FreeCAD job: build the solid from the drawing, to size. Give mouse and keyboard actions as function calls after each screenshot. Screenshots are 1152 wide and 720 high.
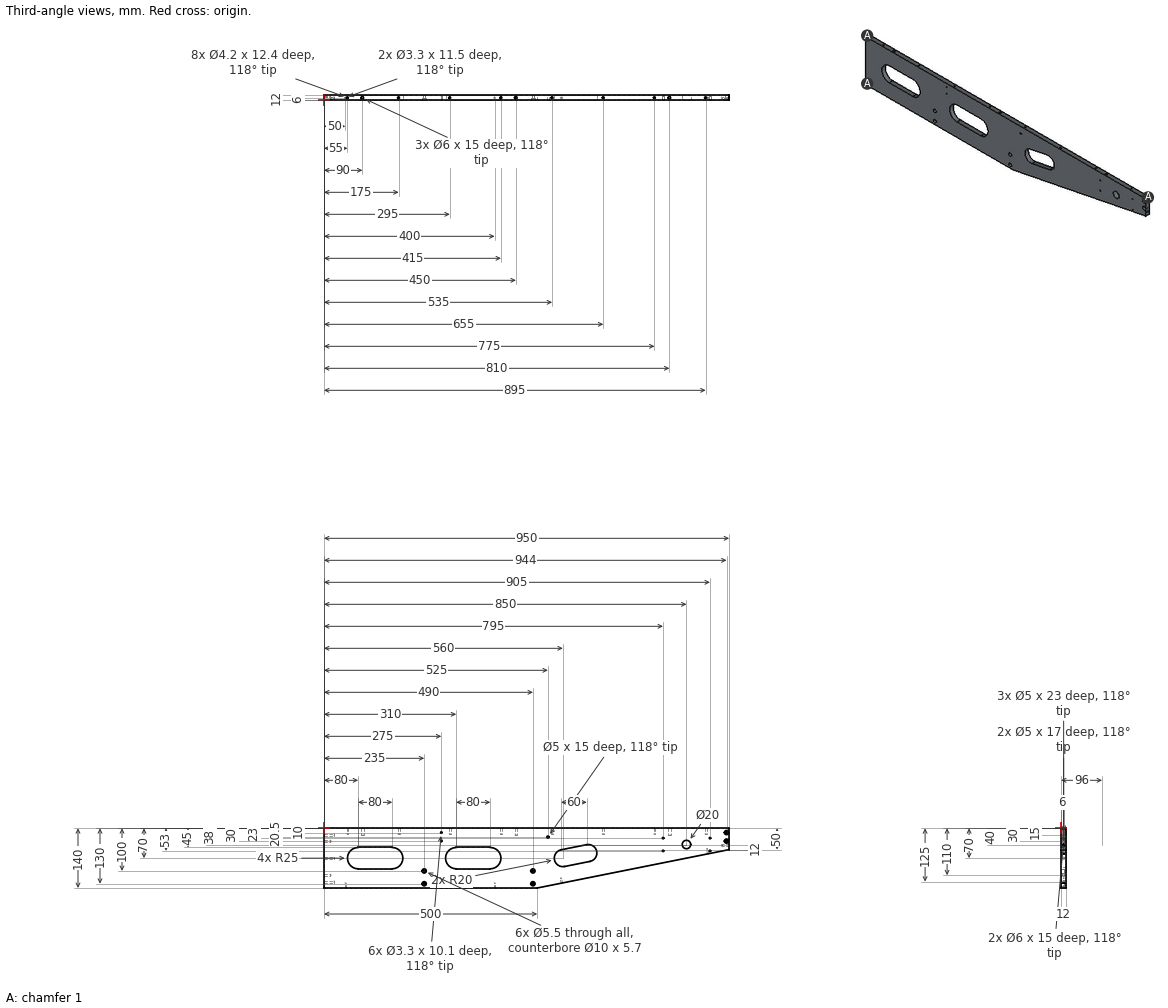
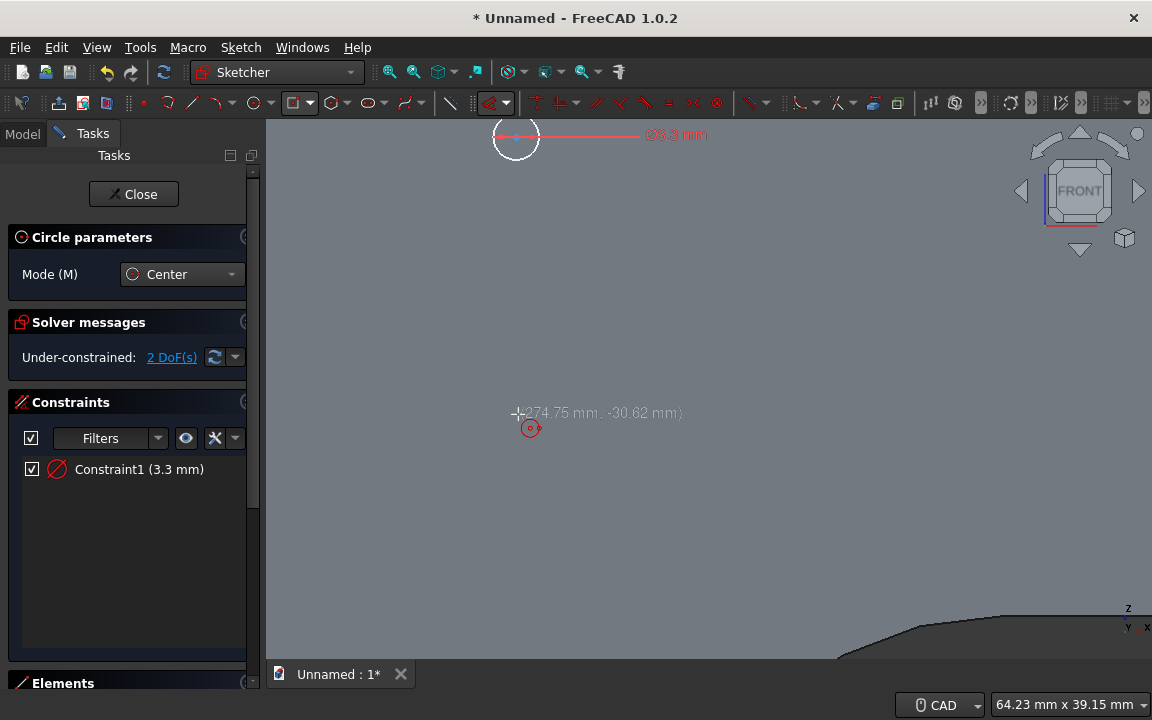
scroll(518, 390, down, 15)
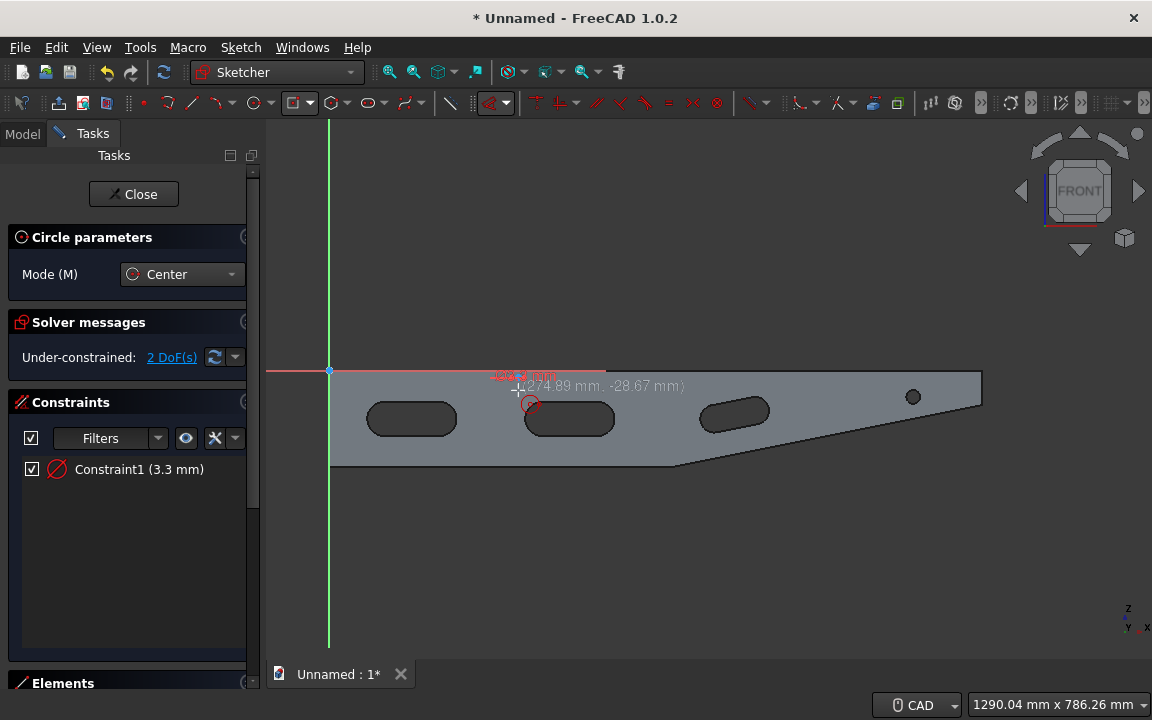
scroll(518, 391, up, 2)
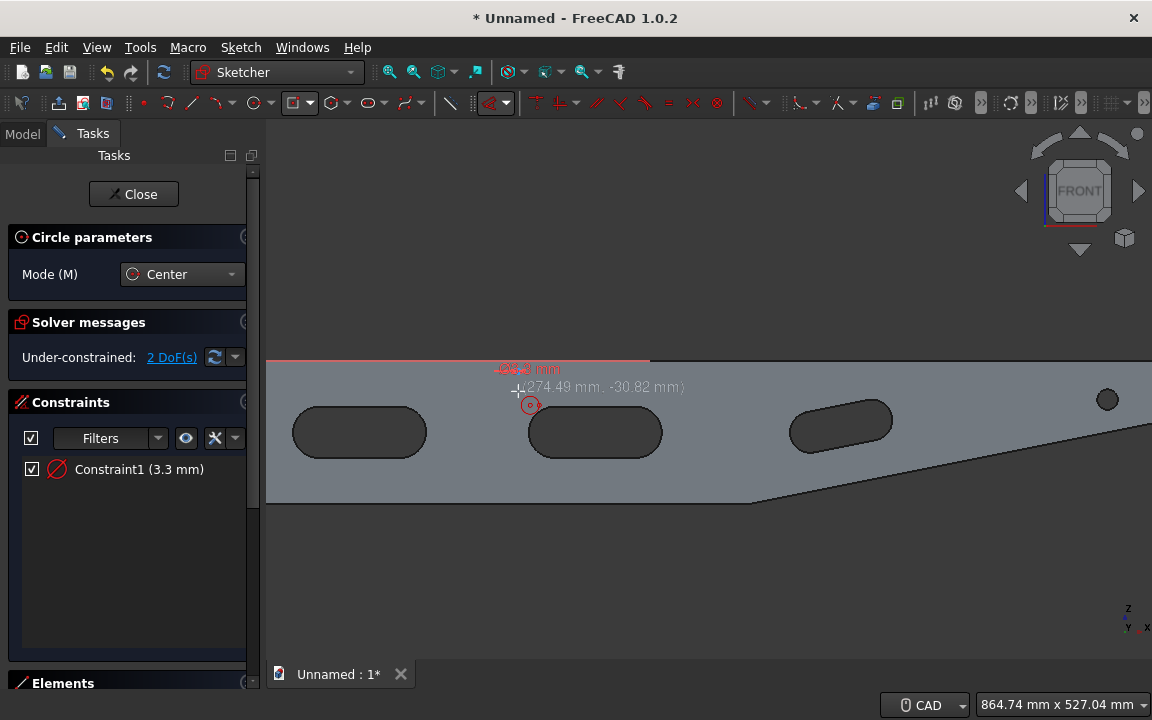
click(518, 391)
move(520, 390)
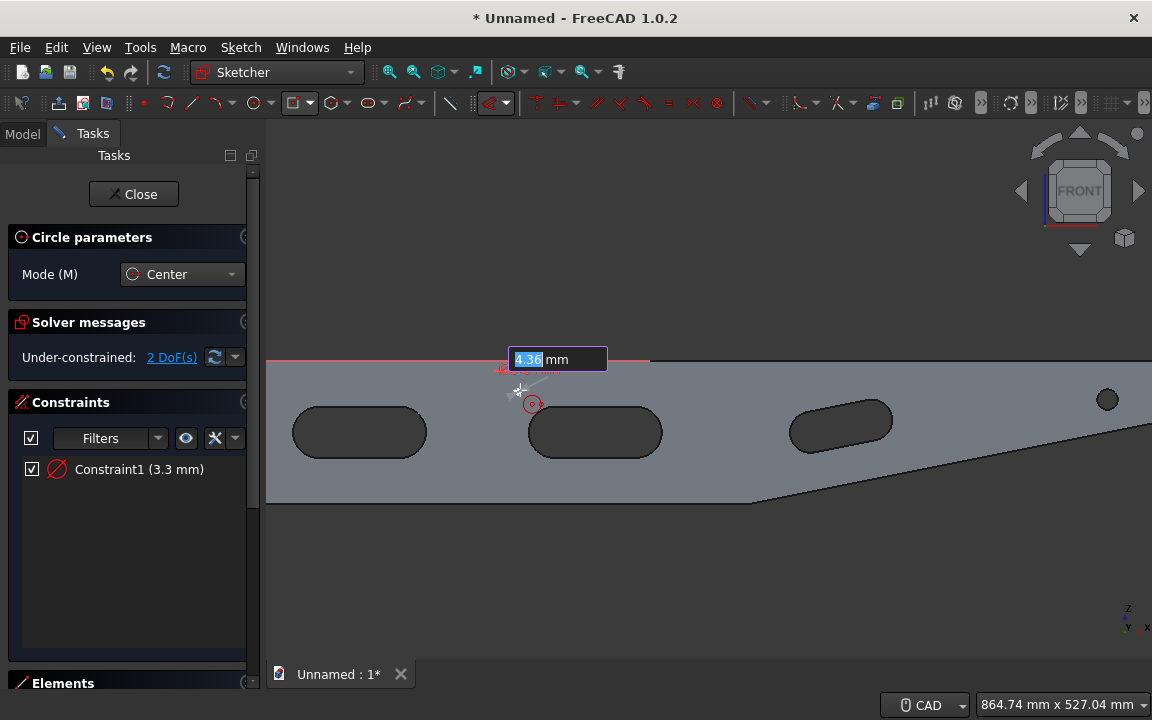
text(3.3)
key(Return)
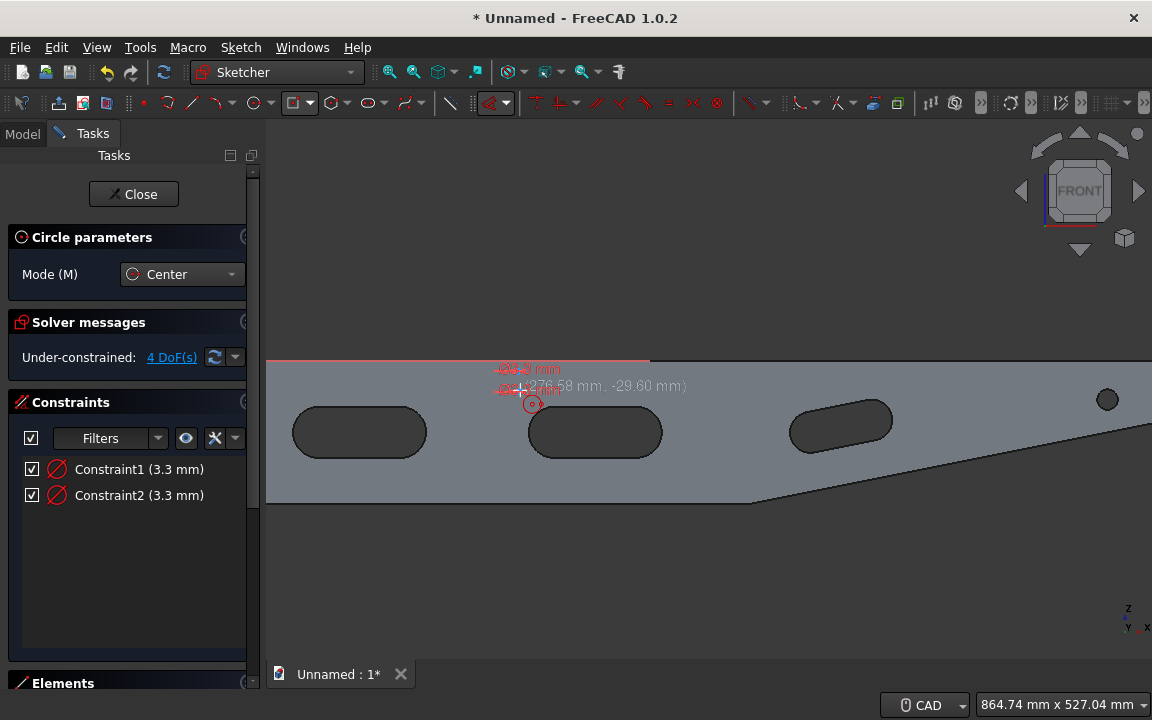
scroll(567, 389, down, 3)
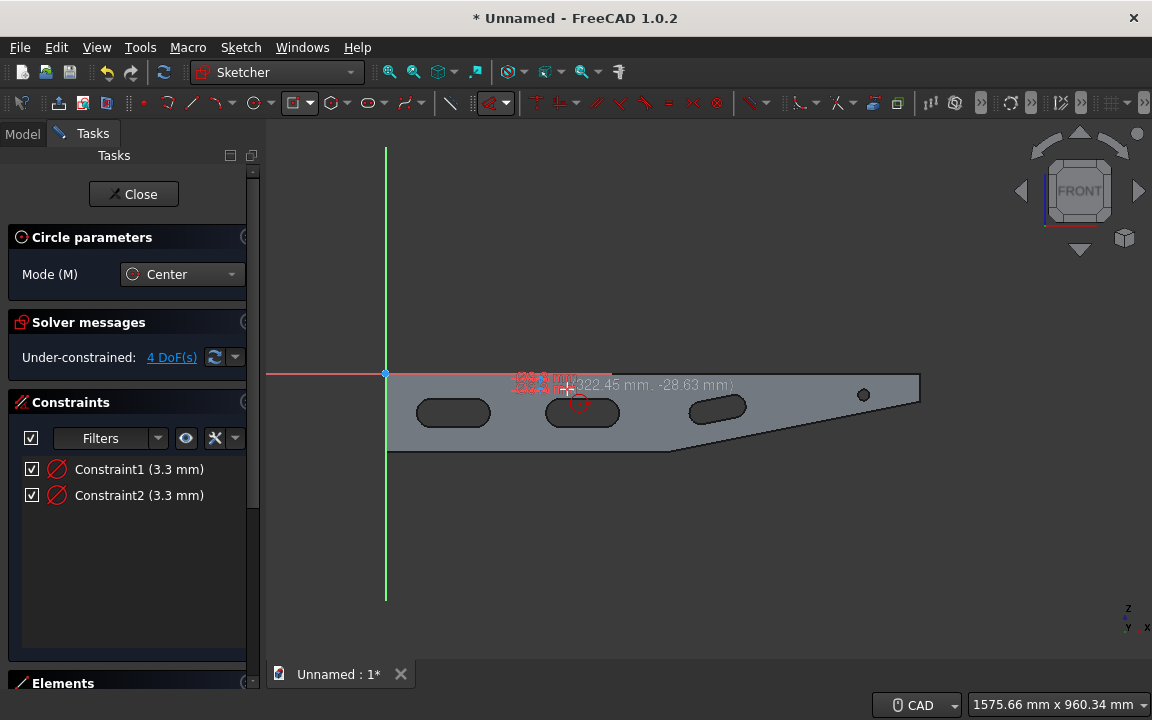
scroll(833, 387, up, 16)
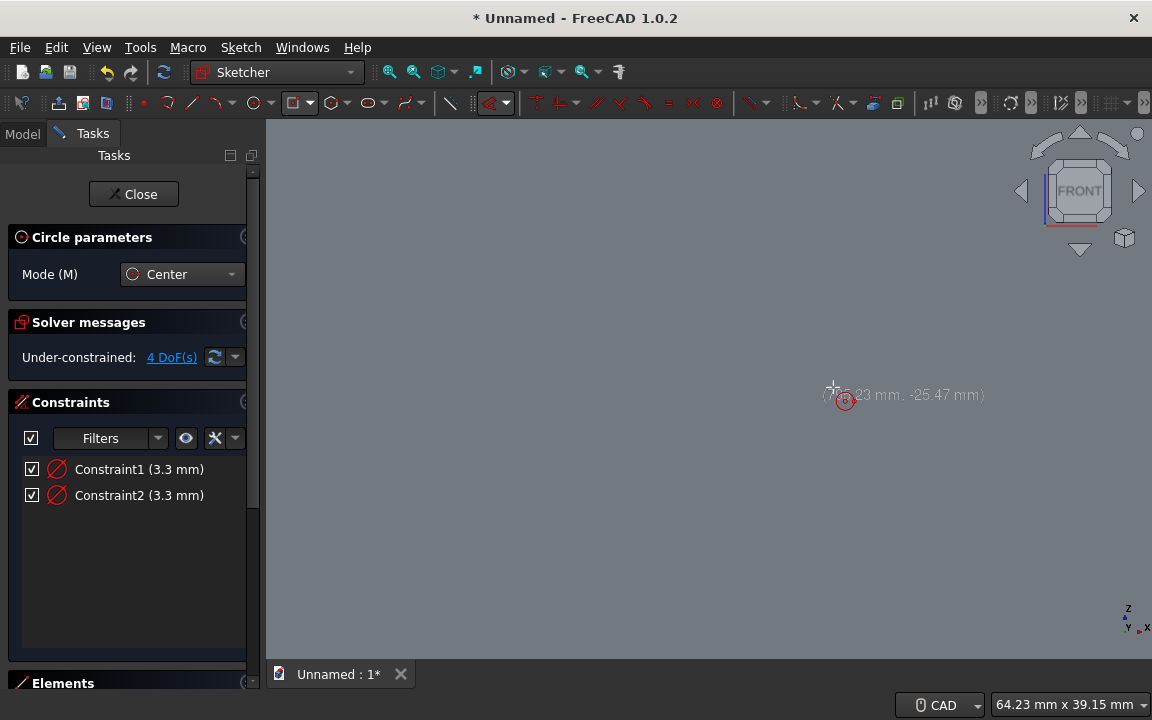
scroll(878, 387, down, 15)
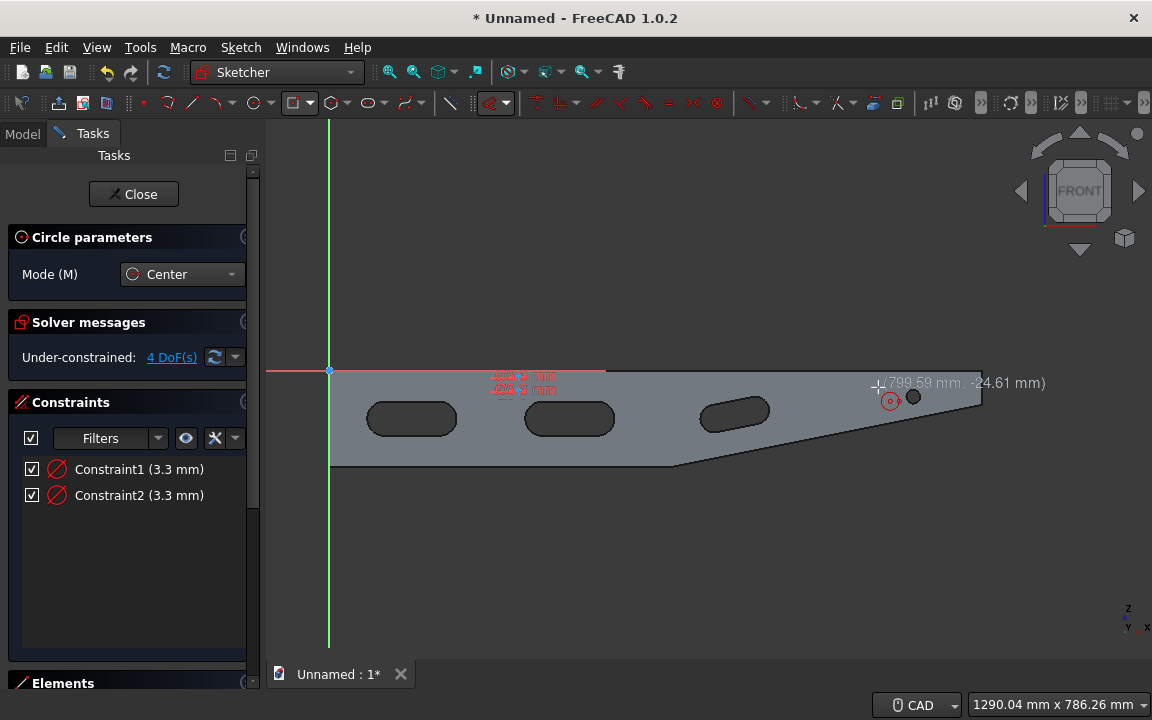
click(876, 386)
move(876, 386)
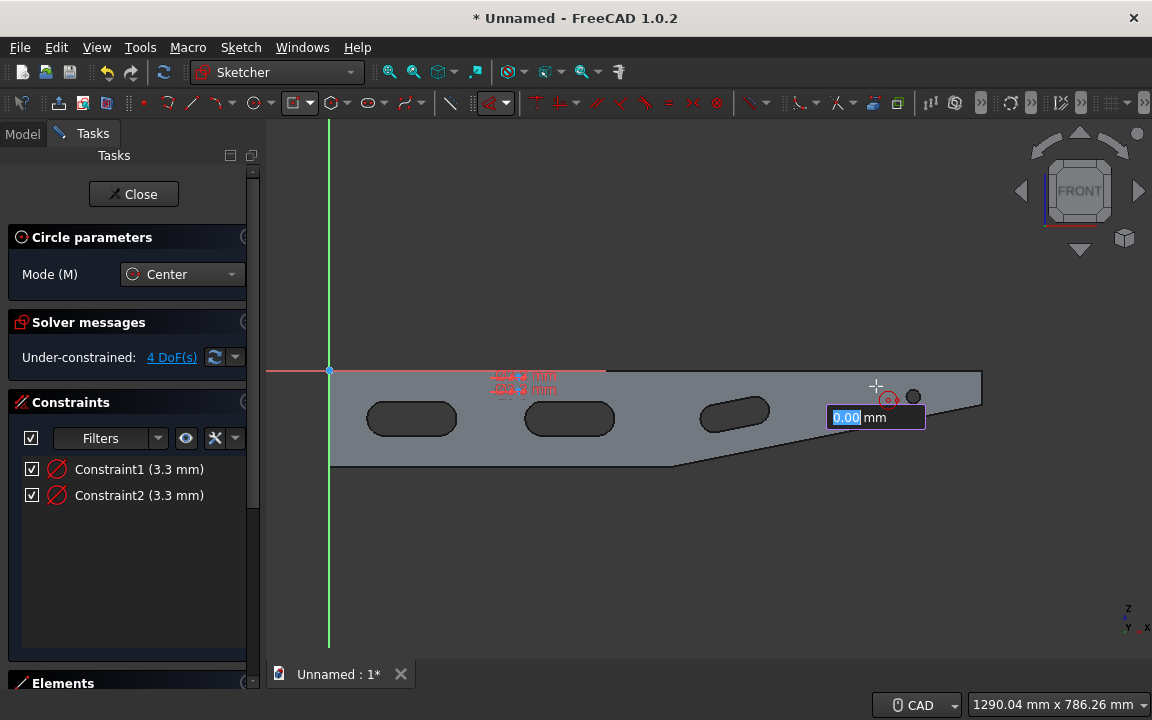
text(3.3)
key(Return)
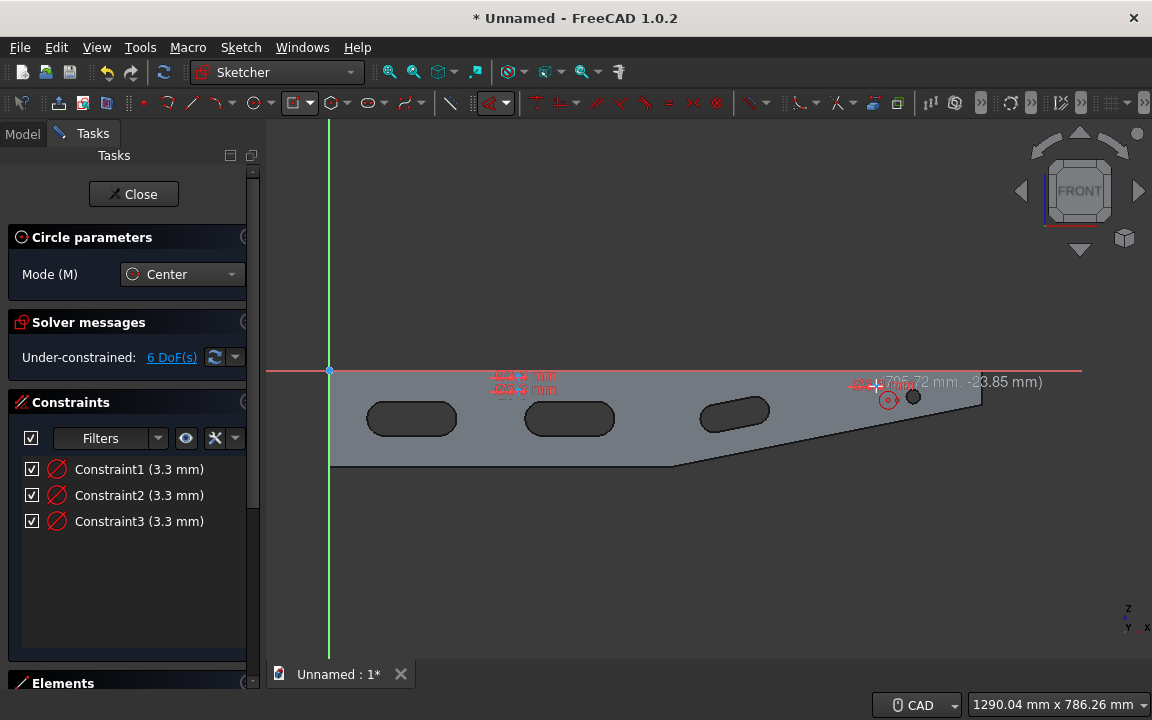
scroll(951, 386, up, 15)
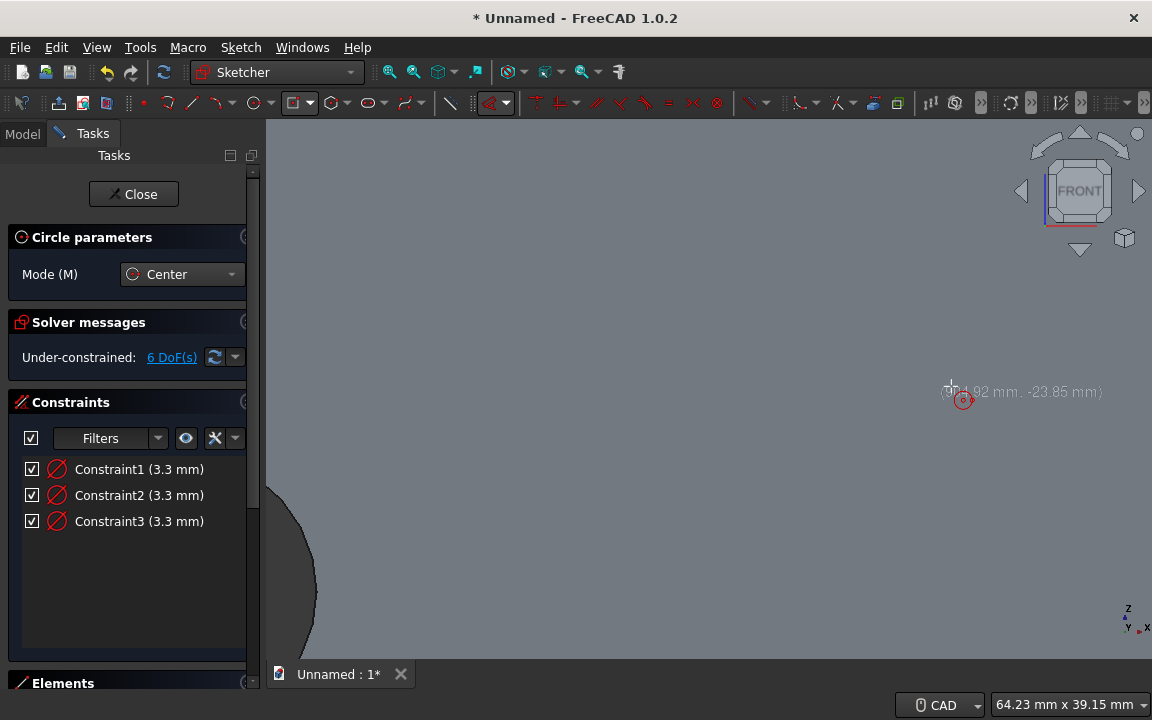
scroll(951, 386, down, 15)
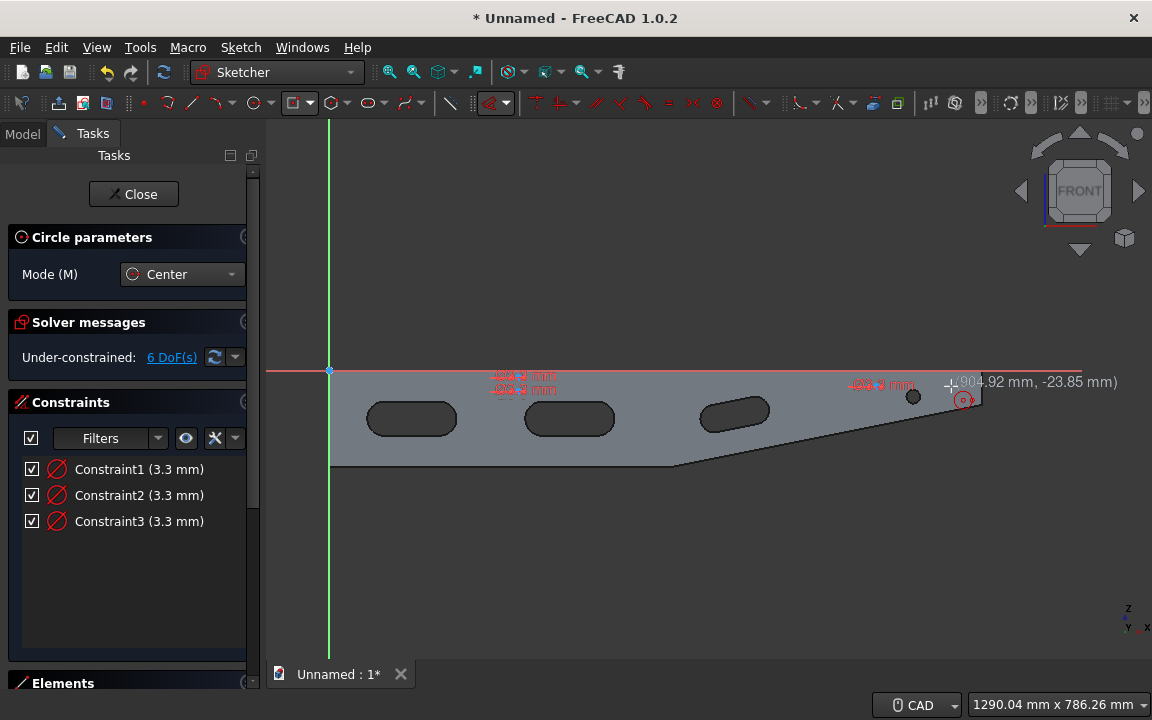
click(951, 386)
move(952, 386)